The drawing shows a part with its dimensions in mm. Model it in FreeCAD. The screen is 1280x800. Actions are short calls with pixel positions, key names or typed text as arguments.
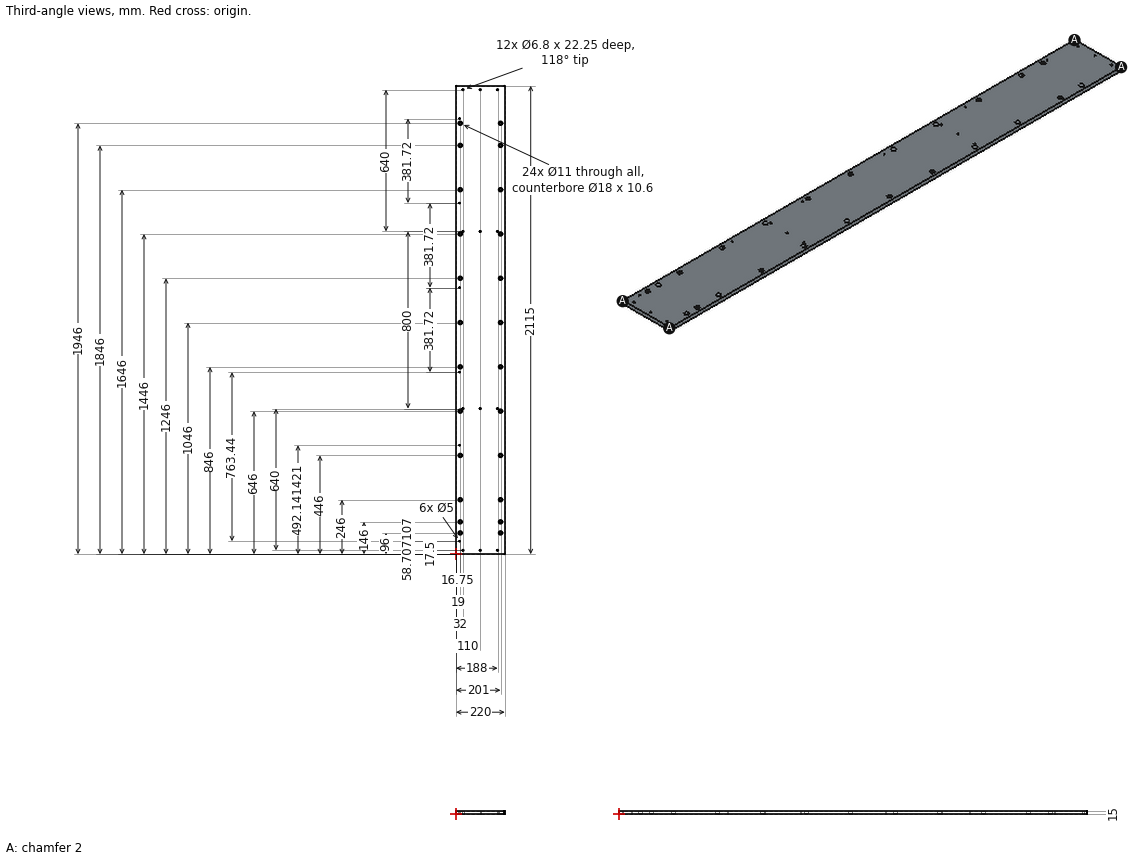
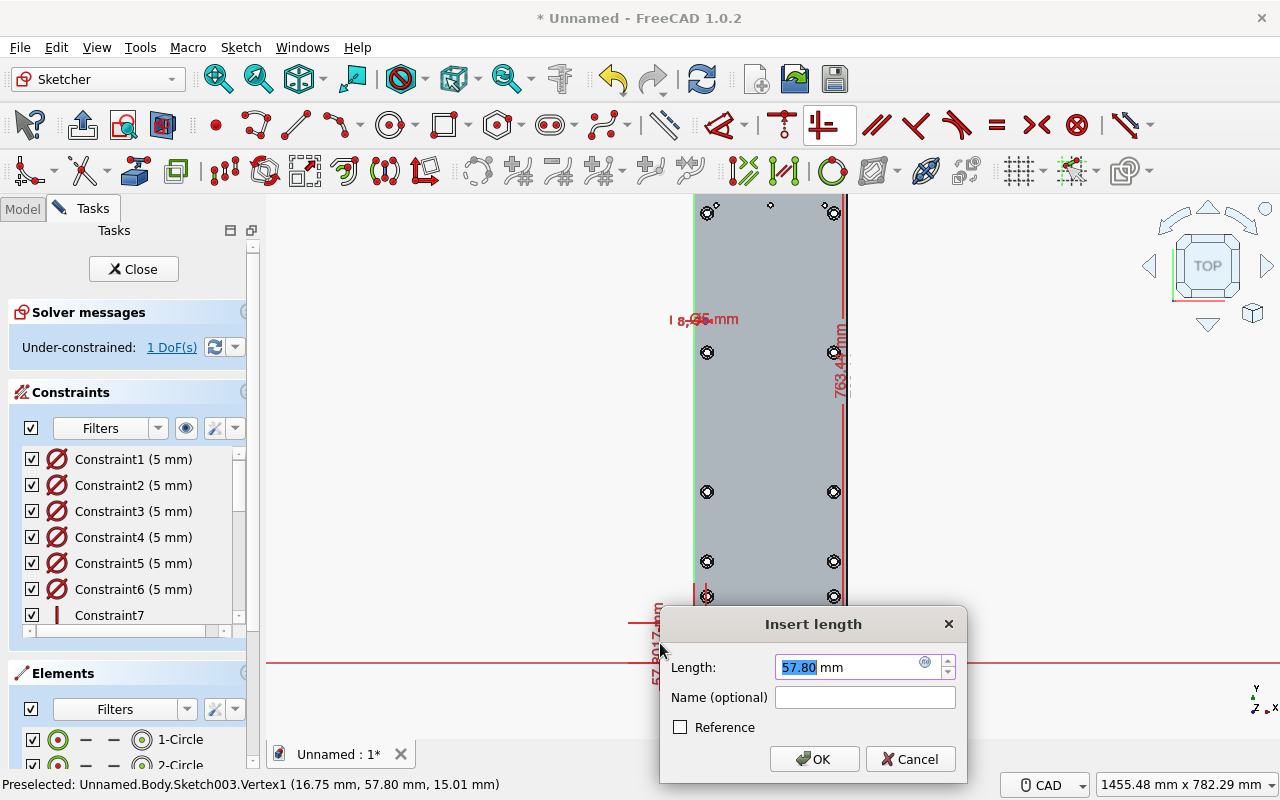
text(58.707107)
key(Return)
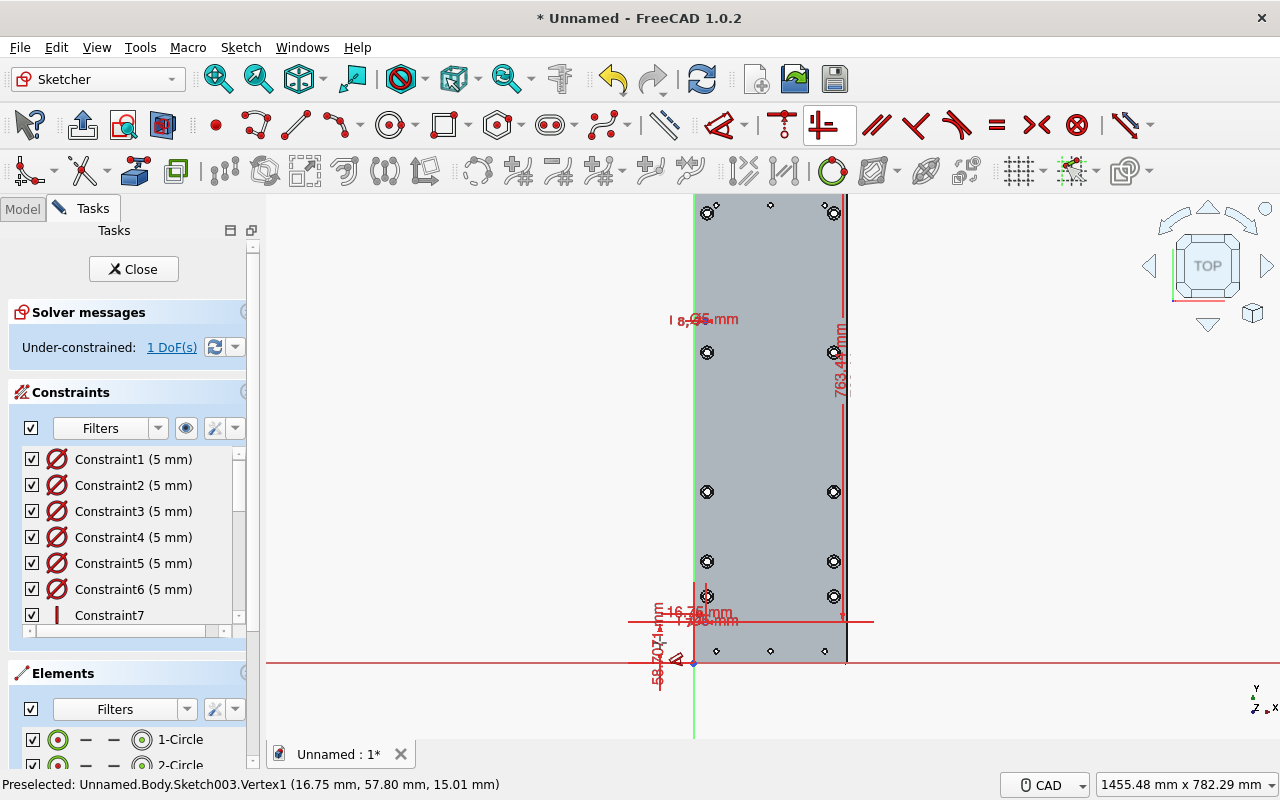
scroll(706, 627, down, 7)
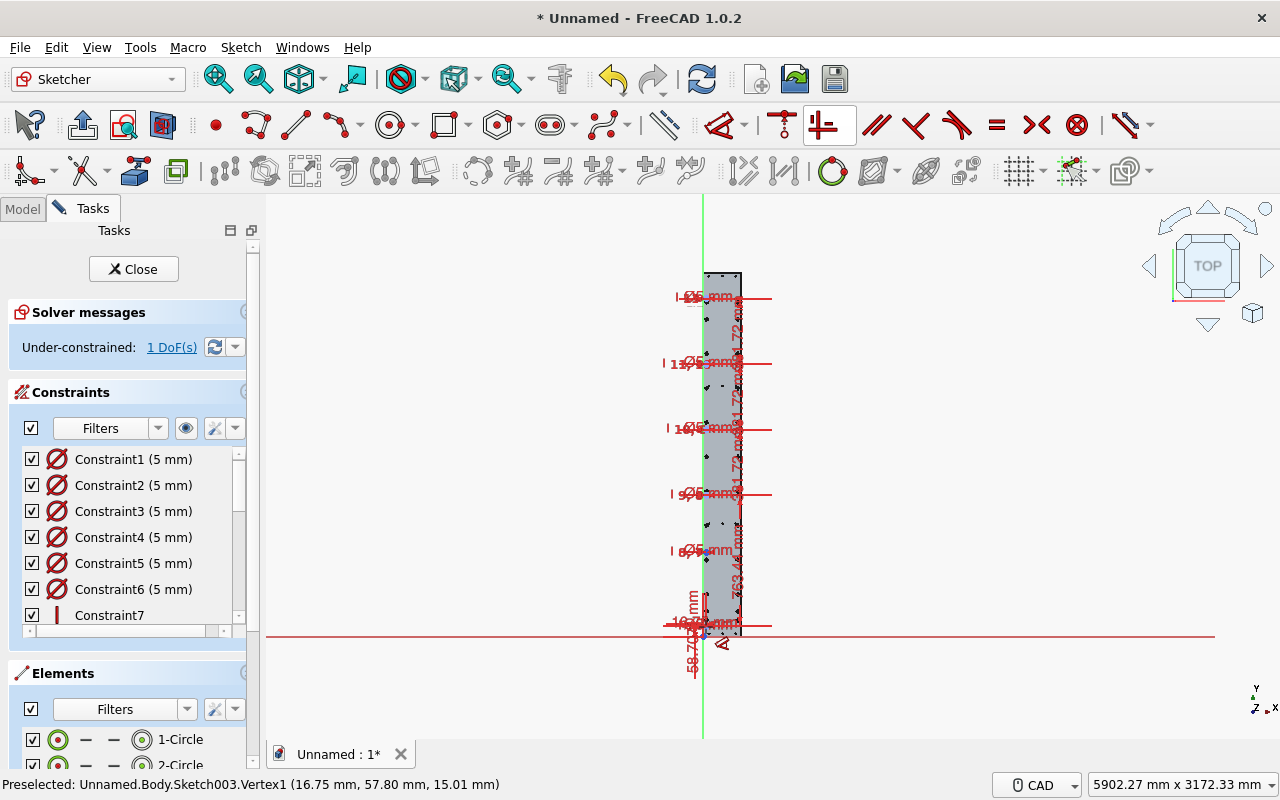
click(706, 552)
click(669, 594)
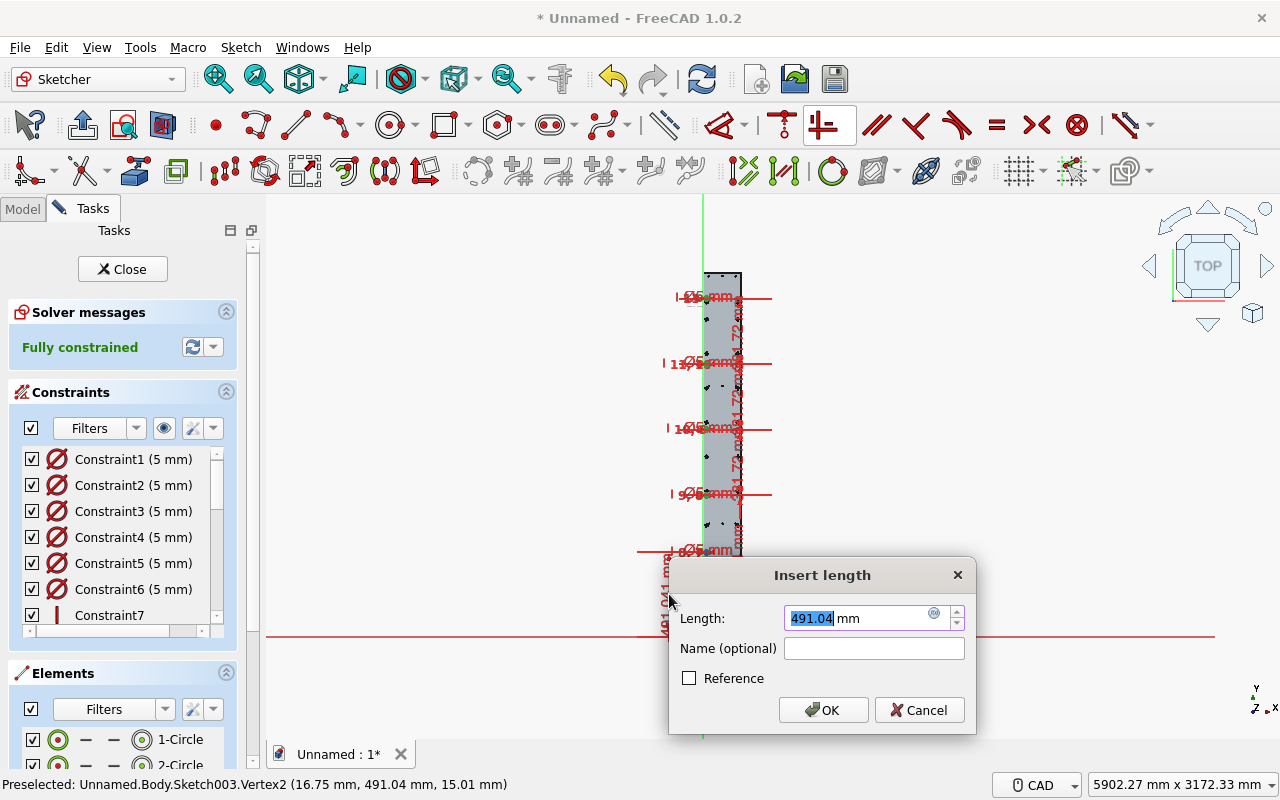
text(492.141421)
key(Return)
key(Escape)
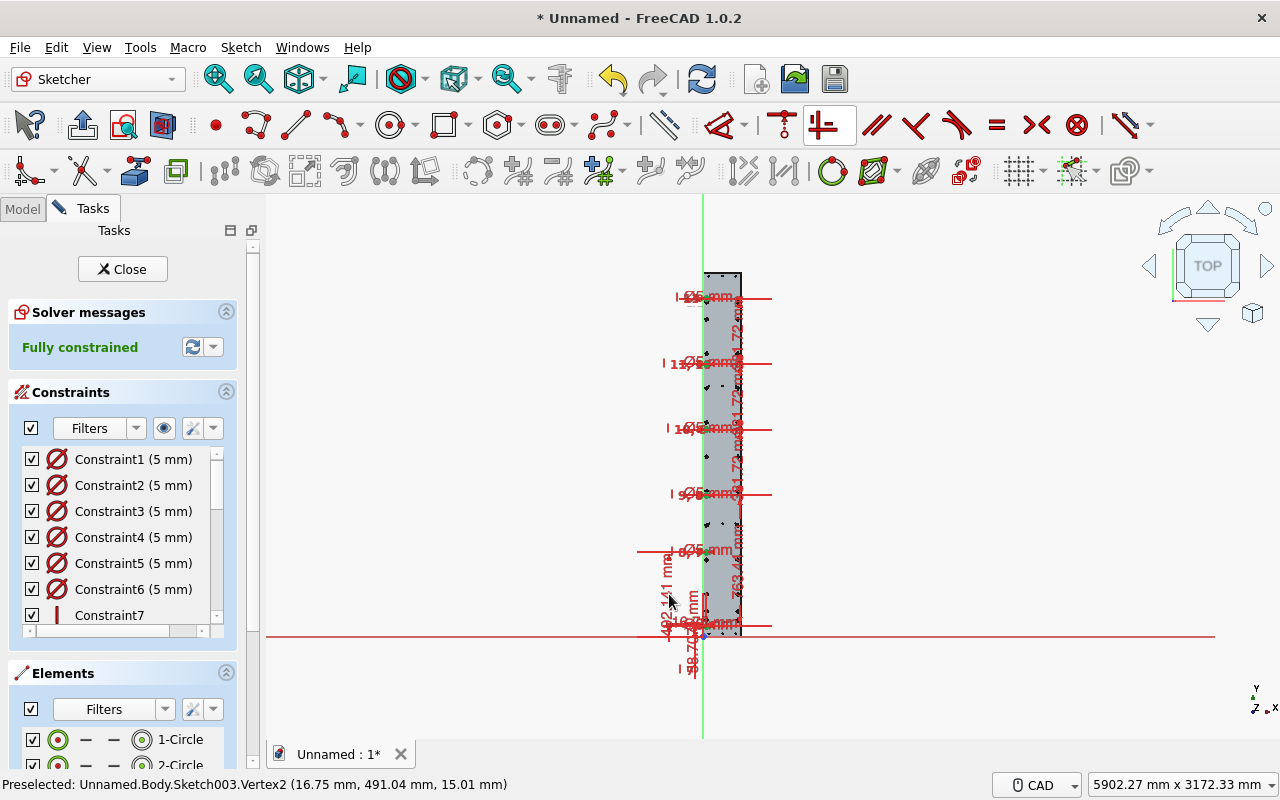
click(123, 269)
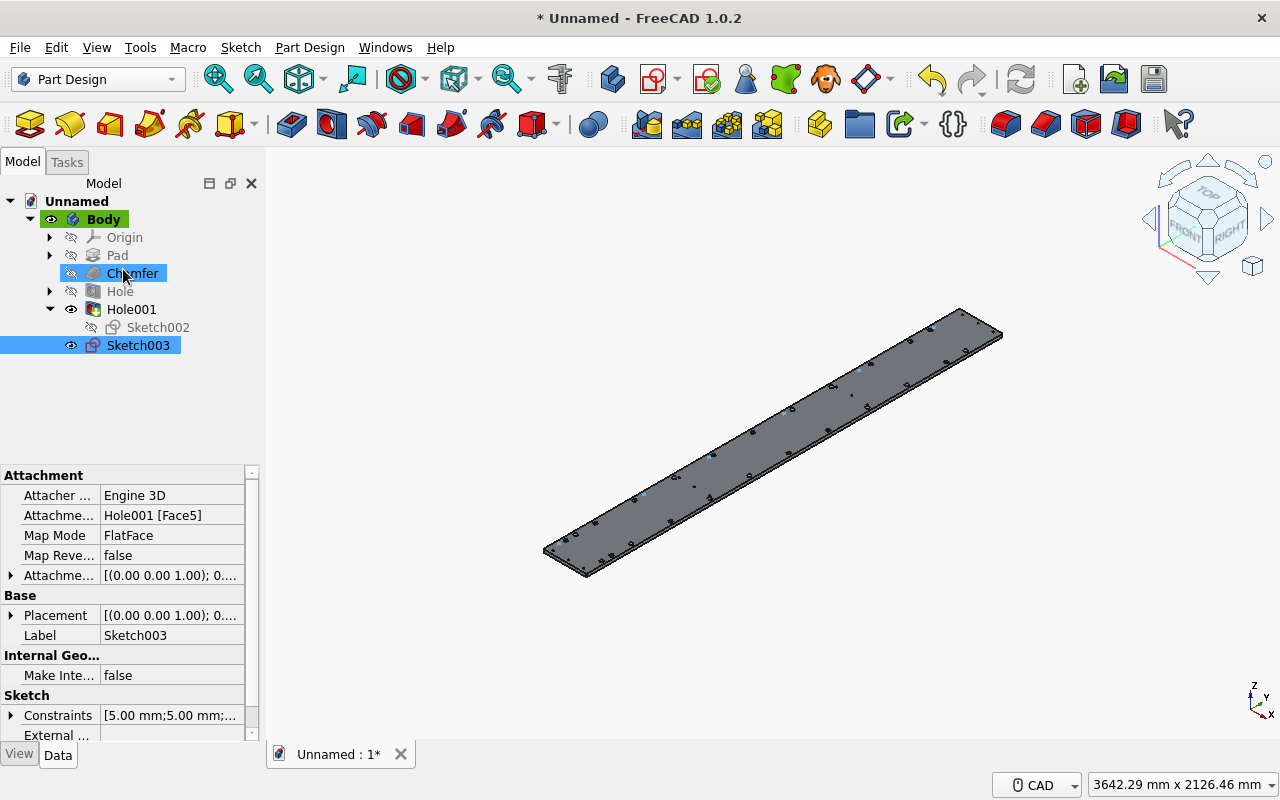
click(292, 124)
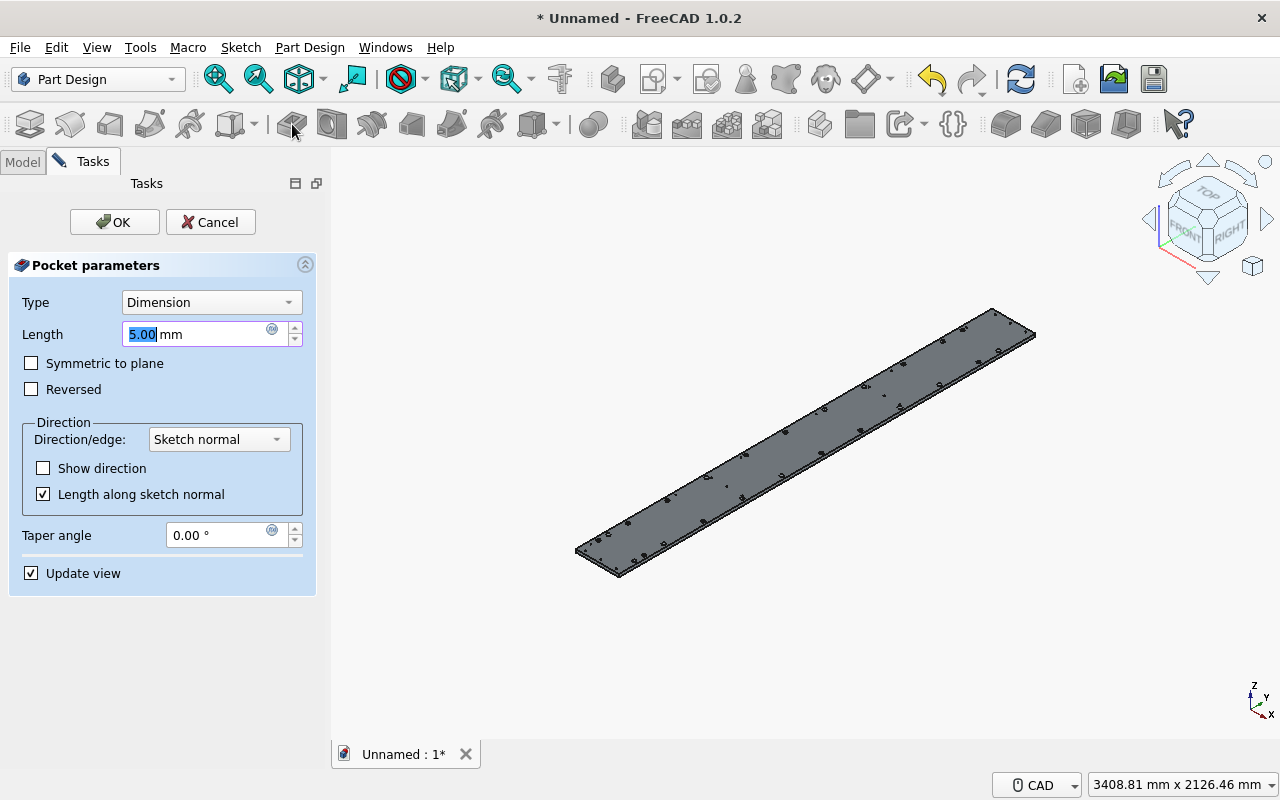
click(212, 302)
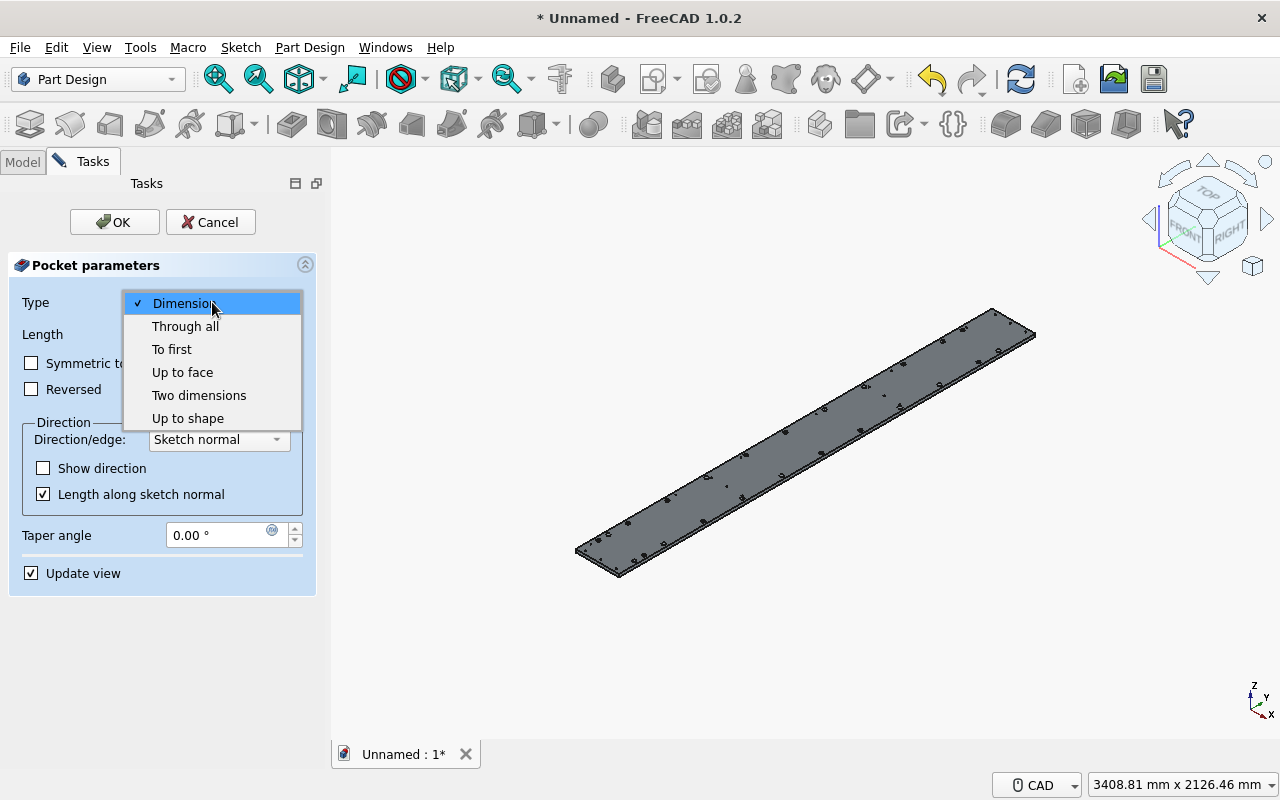
click(212, 326)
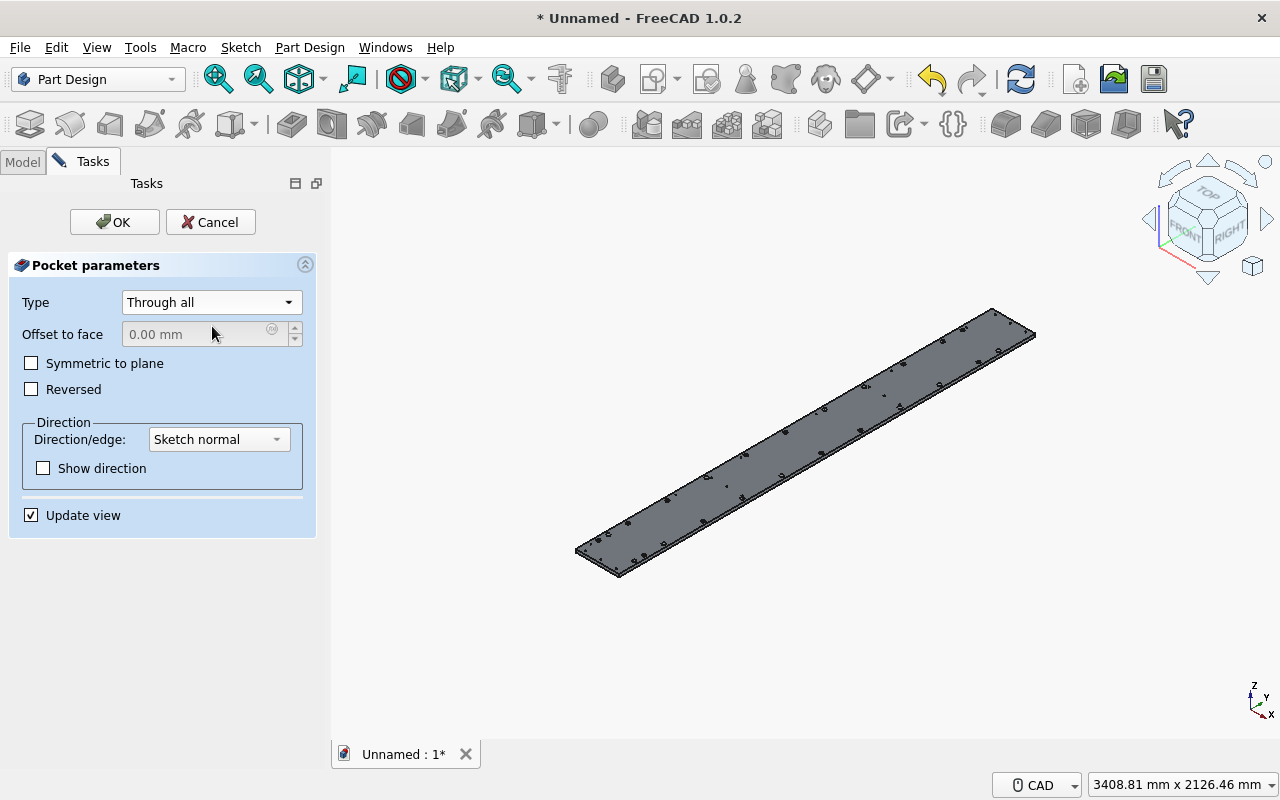
click(115, 222)